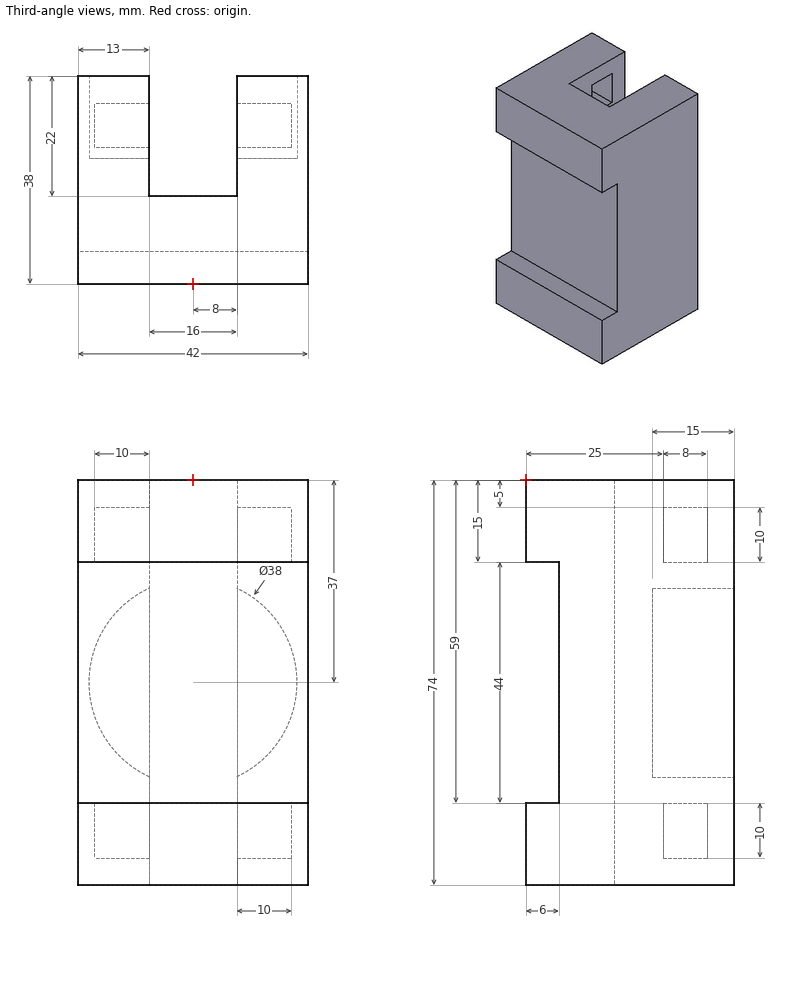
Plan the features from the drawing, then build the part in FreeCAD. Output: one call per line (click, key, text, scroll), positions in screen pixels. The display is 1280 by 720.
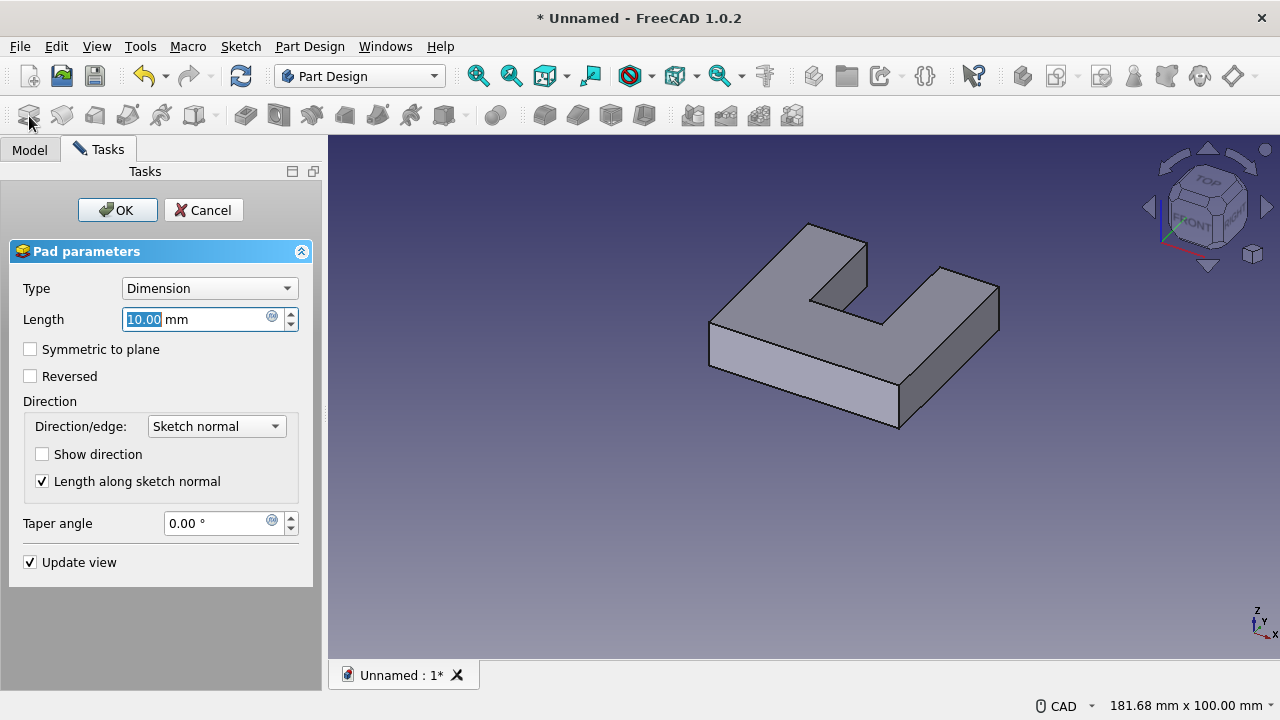
text(74)
key(Tab)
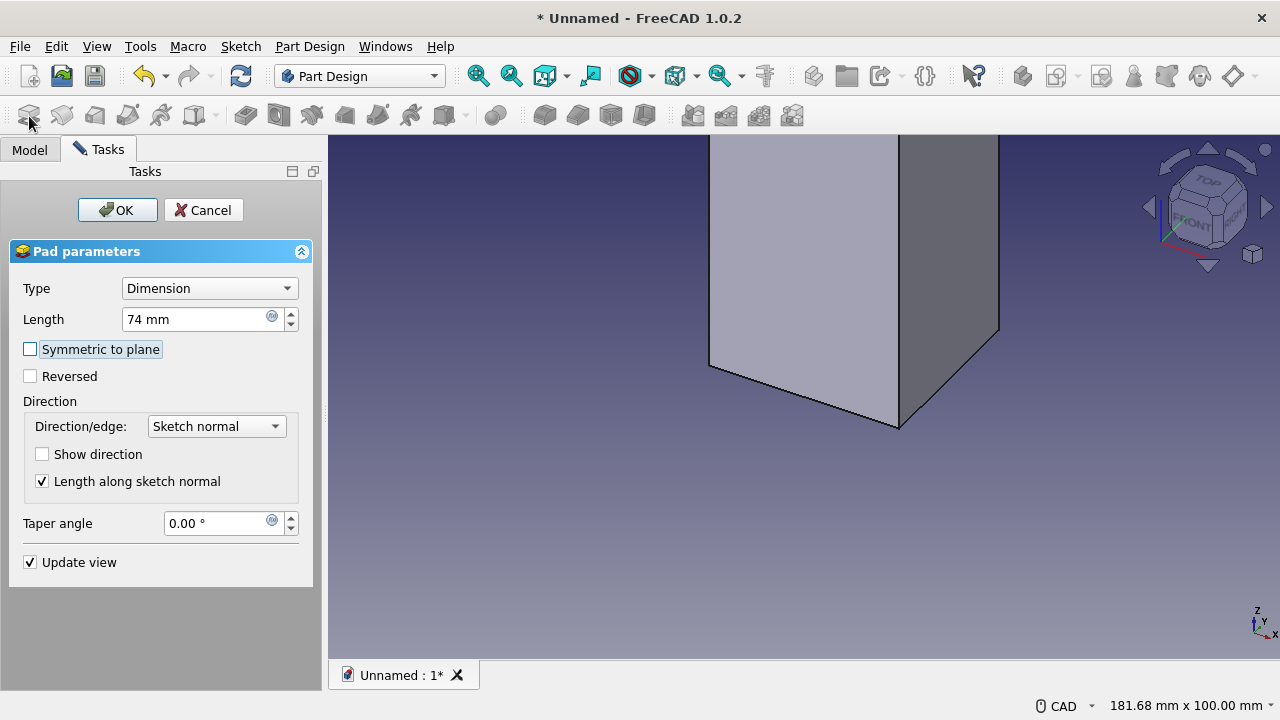
click(31, 376)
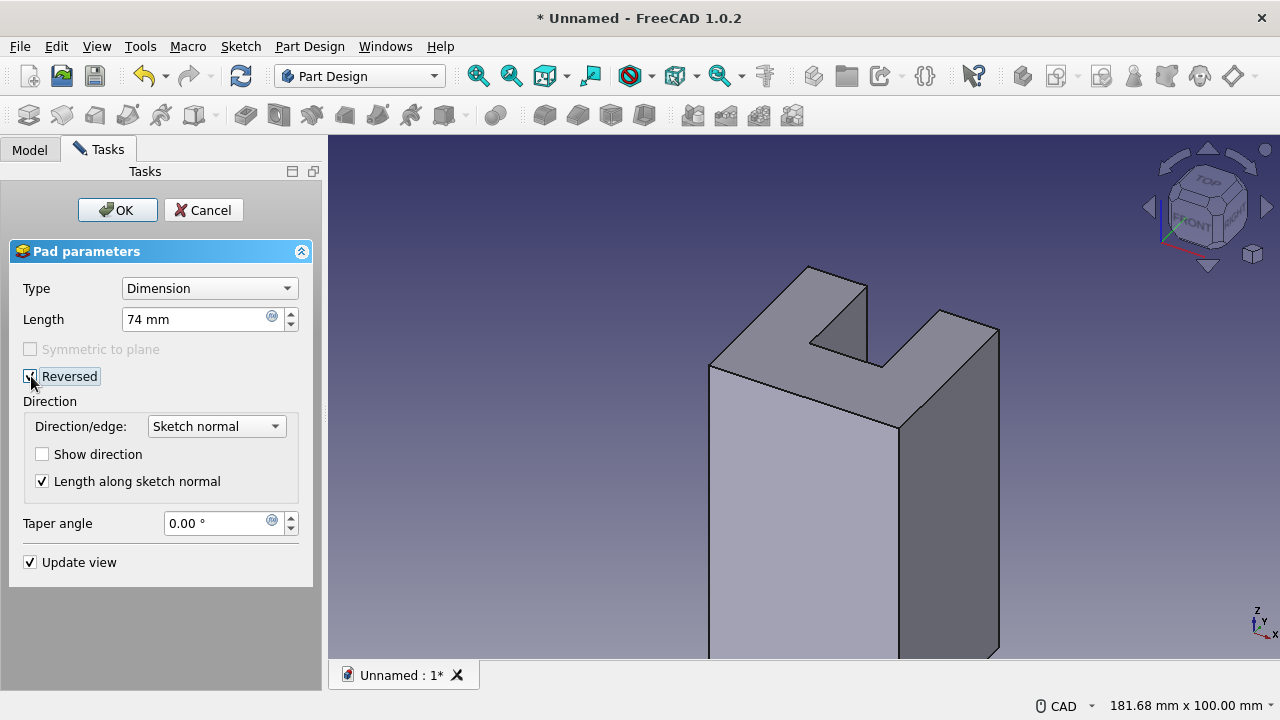
click(118, 210)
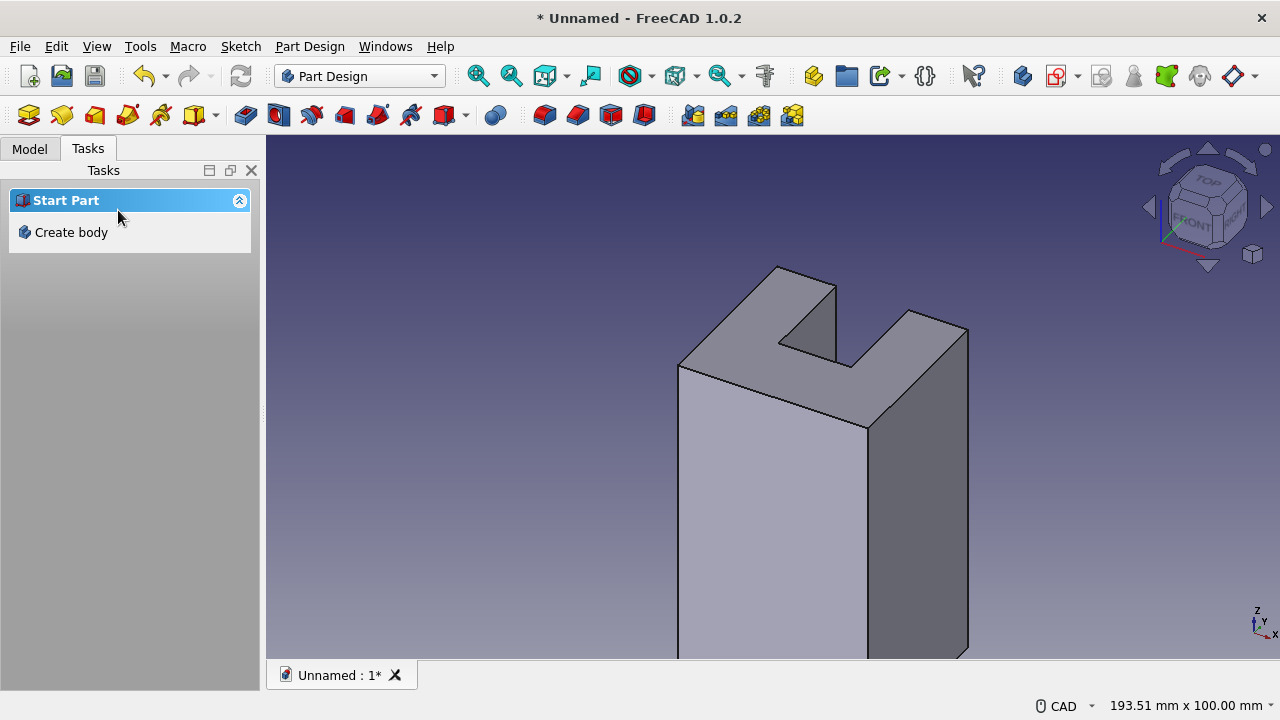
key(v)
key(f)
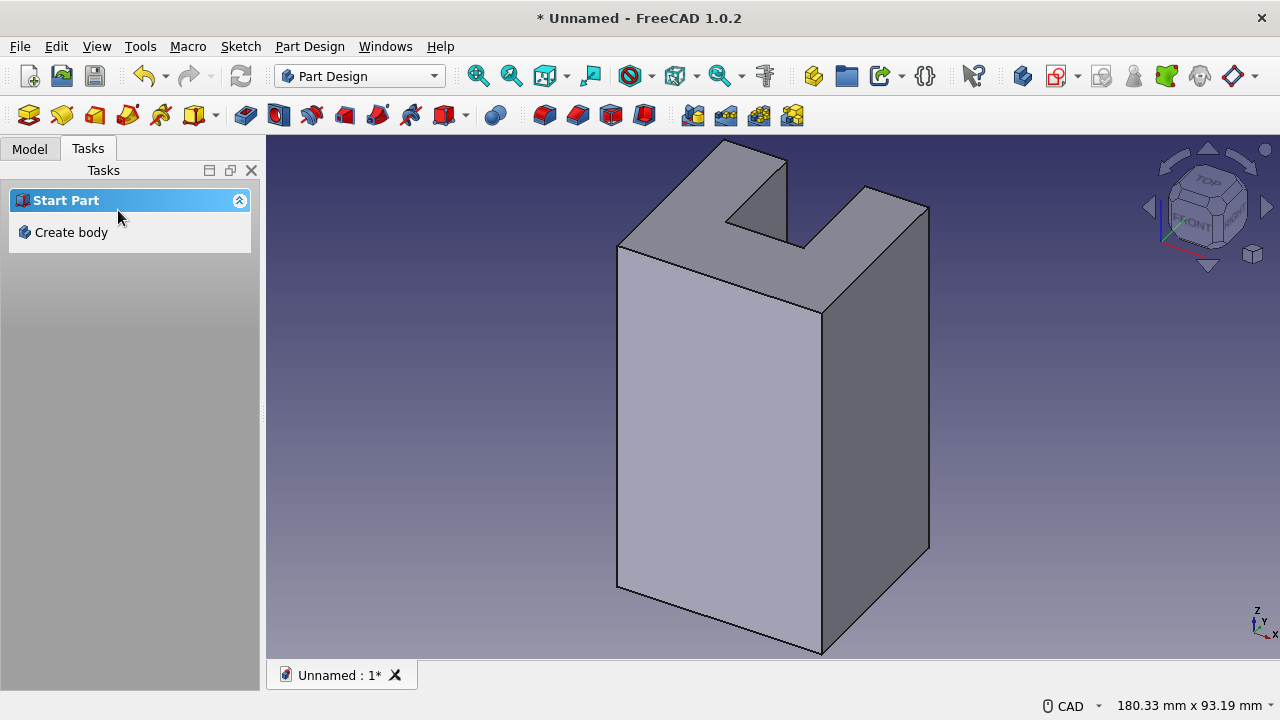
click(875, 381)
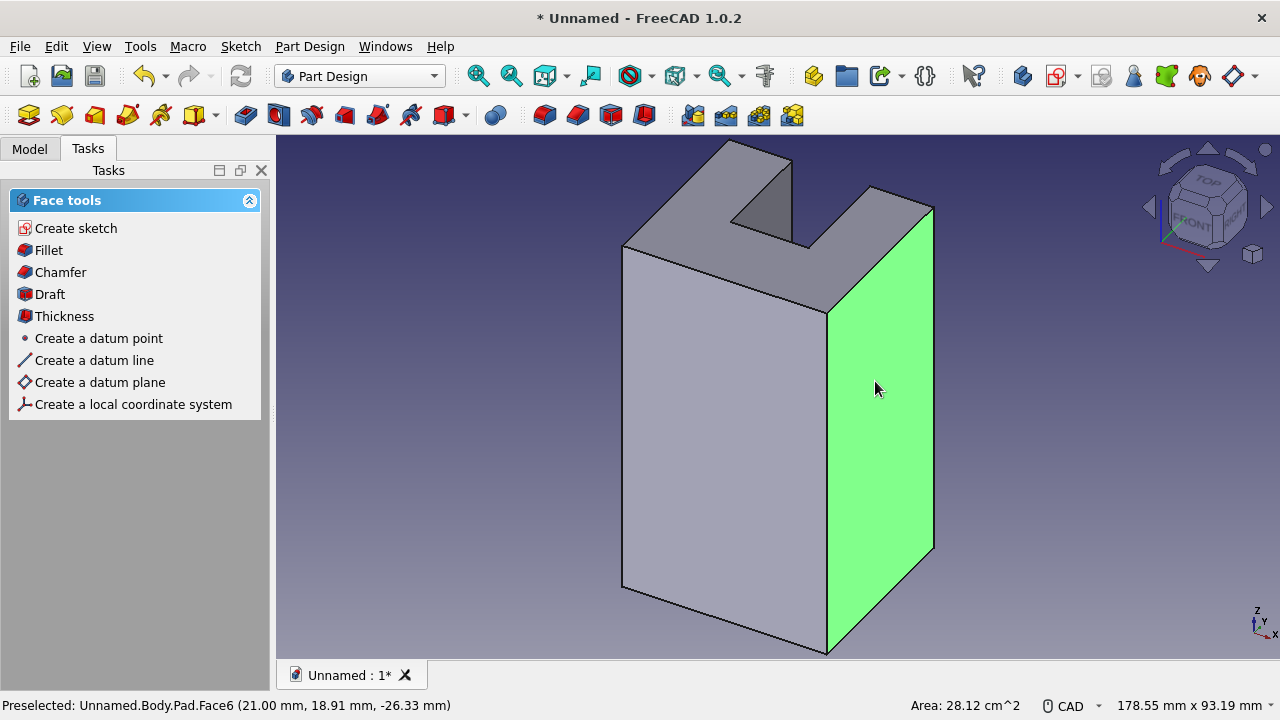
click(1056, 76)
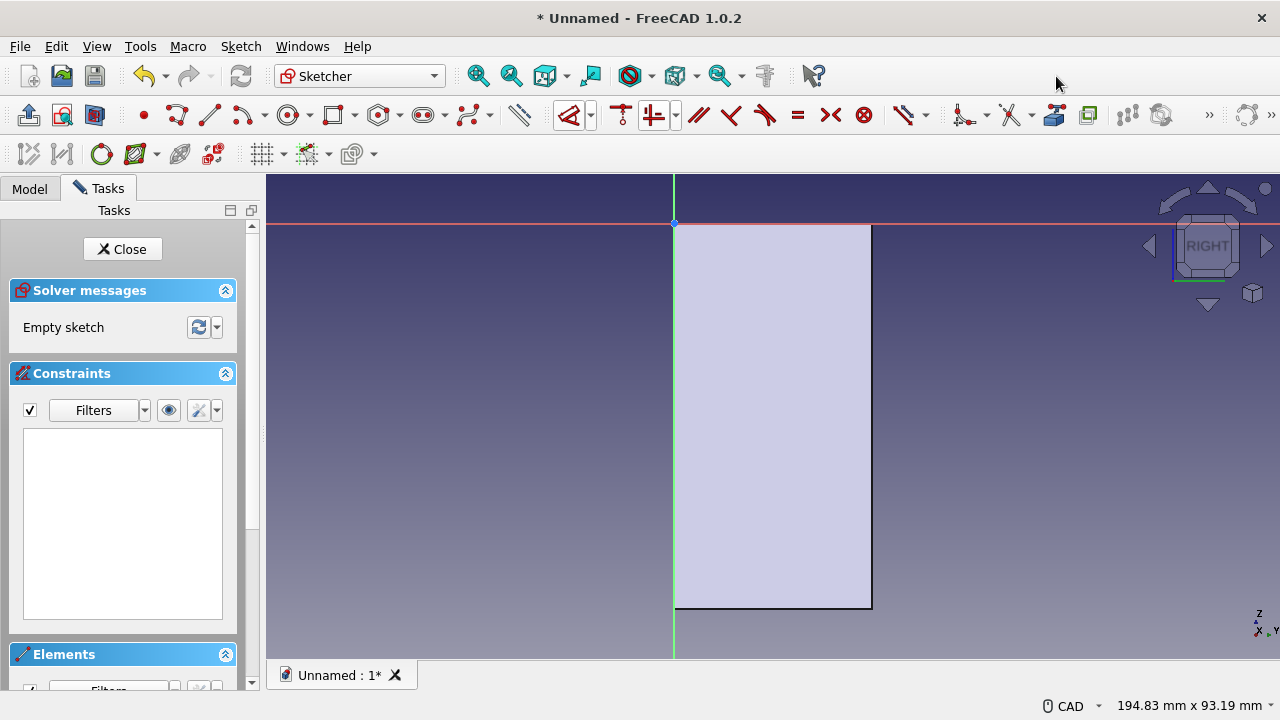
scroll(771, 593, down, 1)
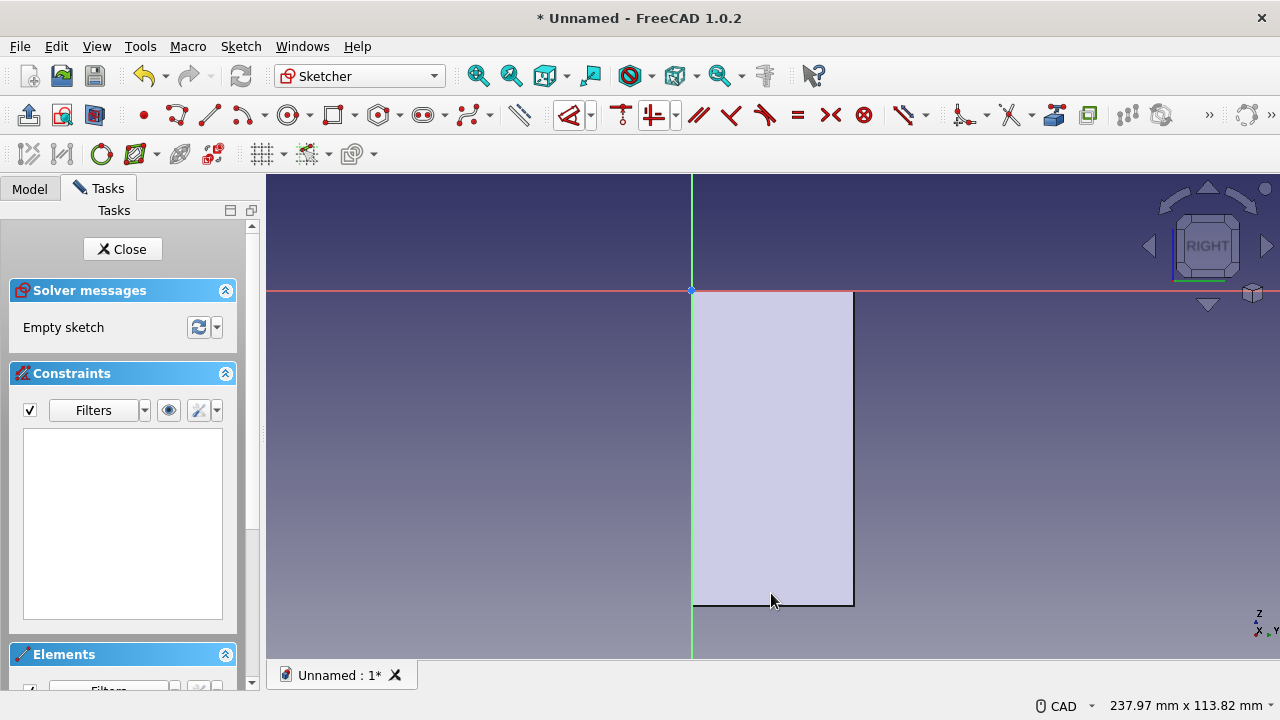
key(g)
key(r)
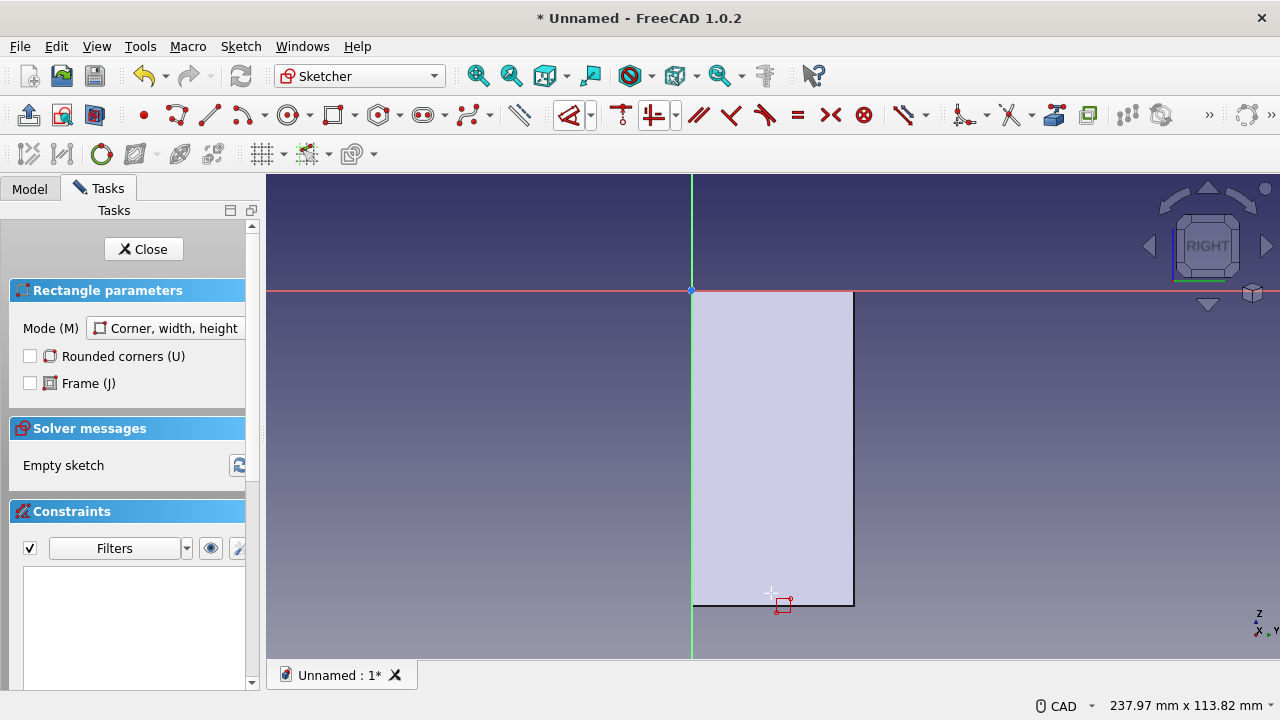
click(692, 355)
move(717, 542)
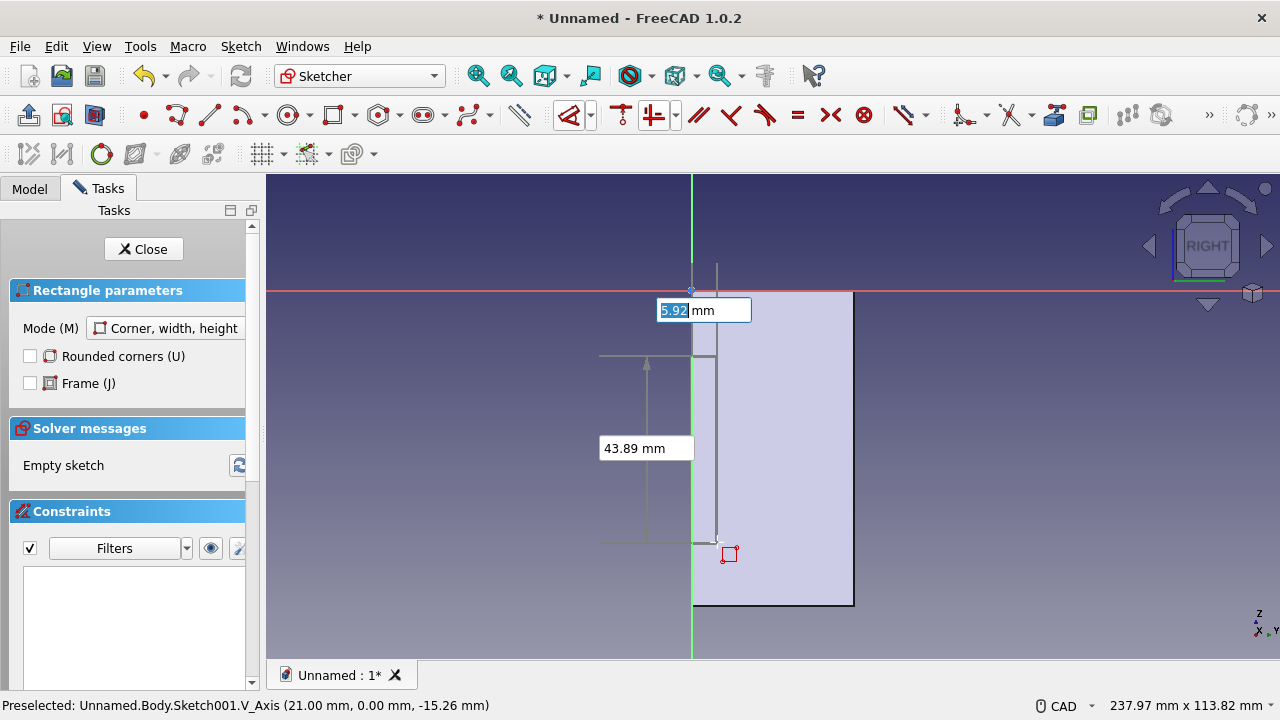
text(6)
key(Tab)
text(44)
key(Return)
key(Escape)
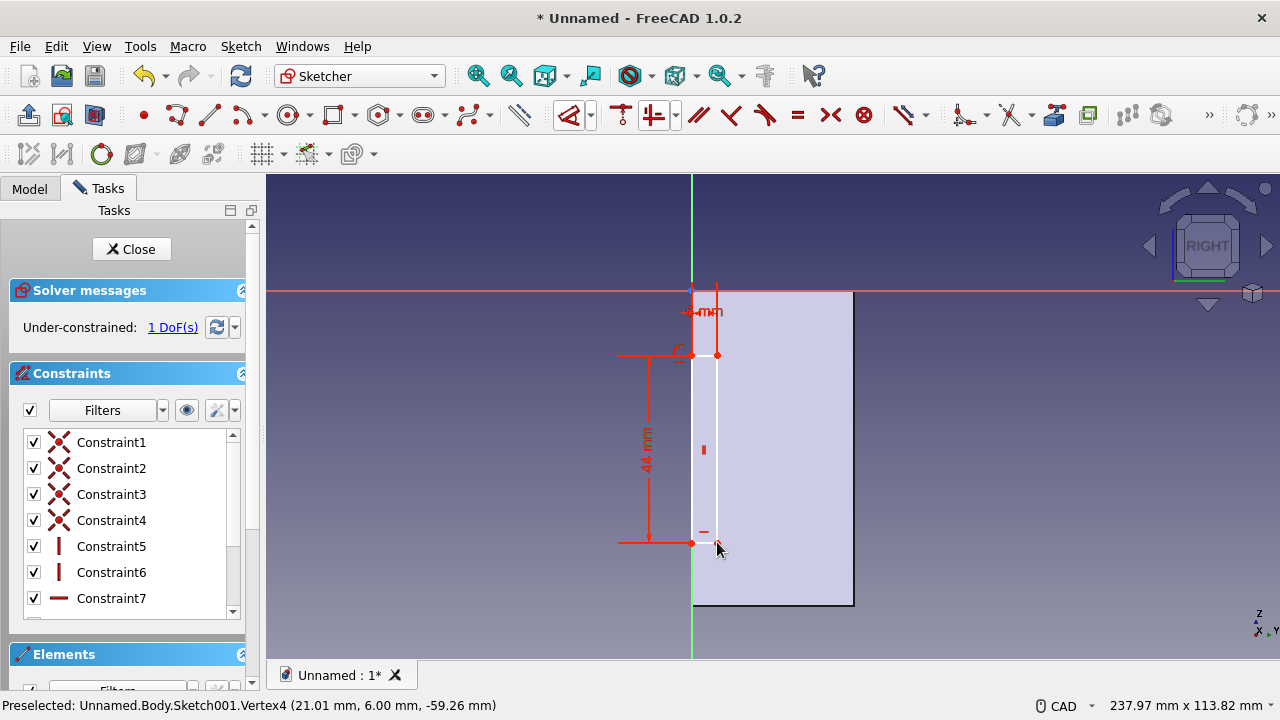
click(692, 356)